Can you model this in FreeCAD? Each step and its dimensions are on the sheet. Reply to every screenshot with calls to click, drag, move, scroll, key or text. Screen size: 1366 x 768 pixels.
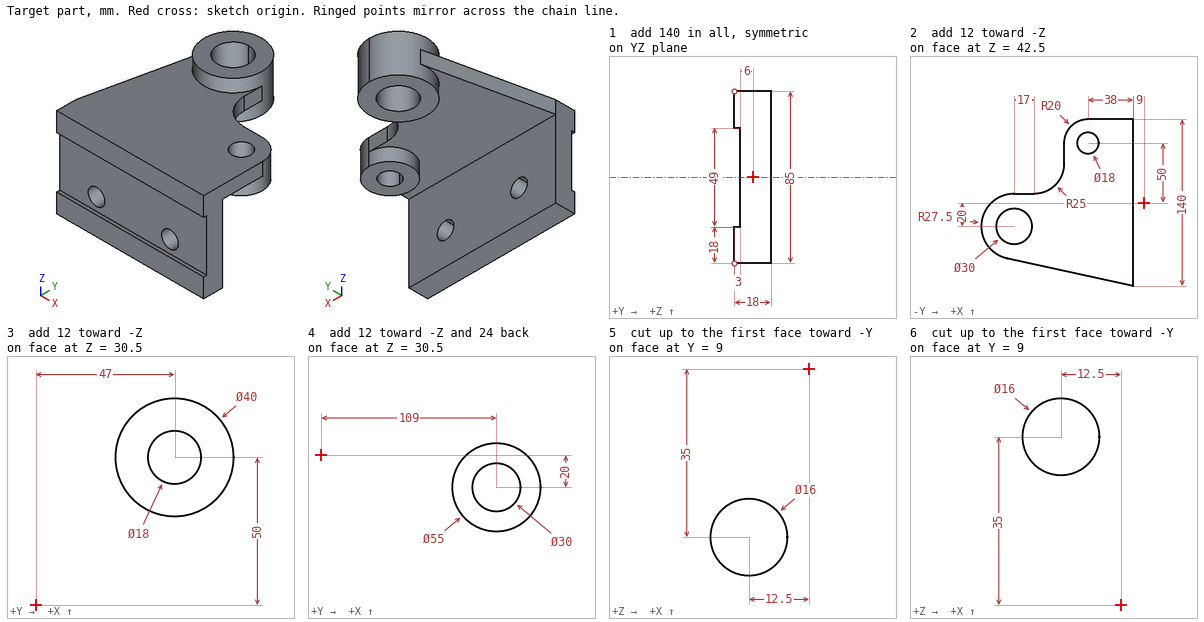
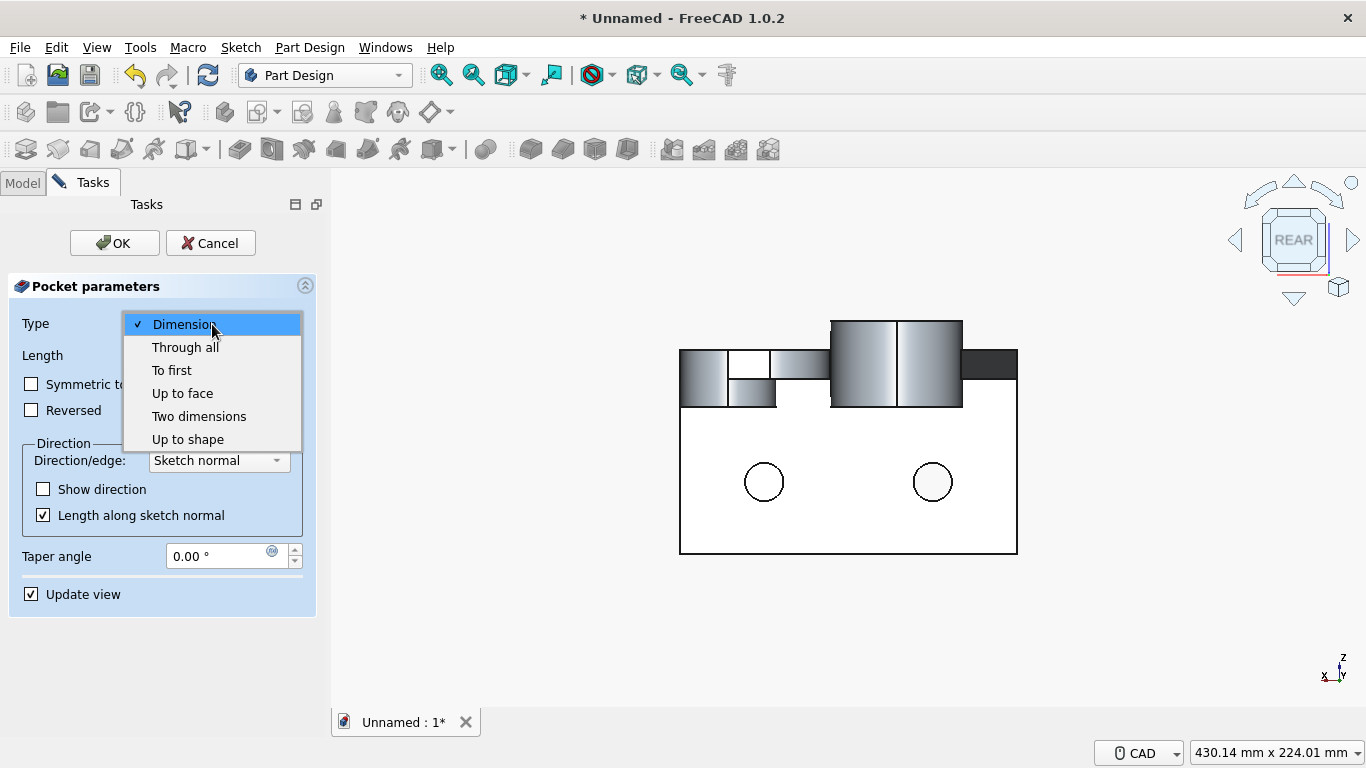
click(212, 370)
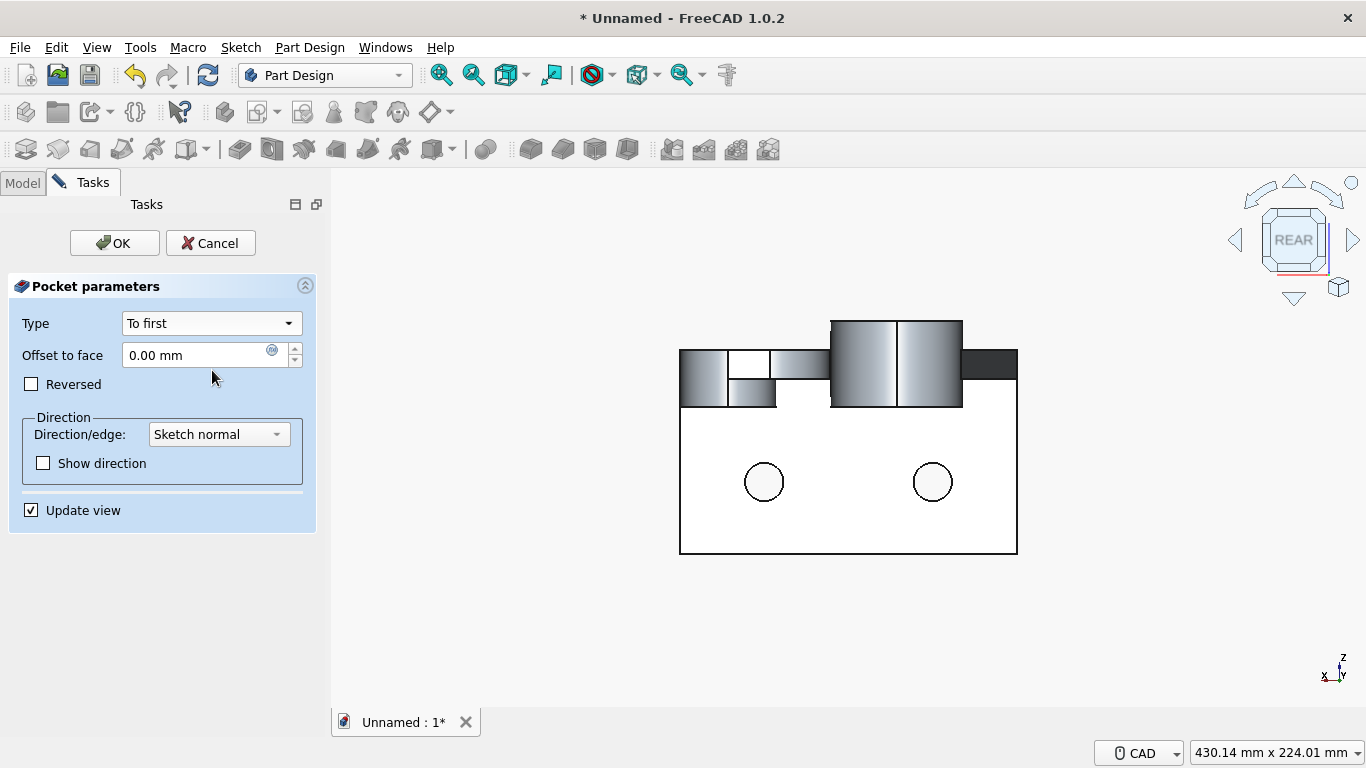
click(115, 243)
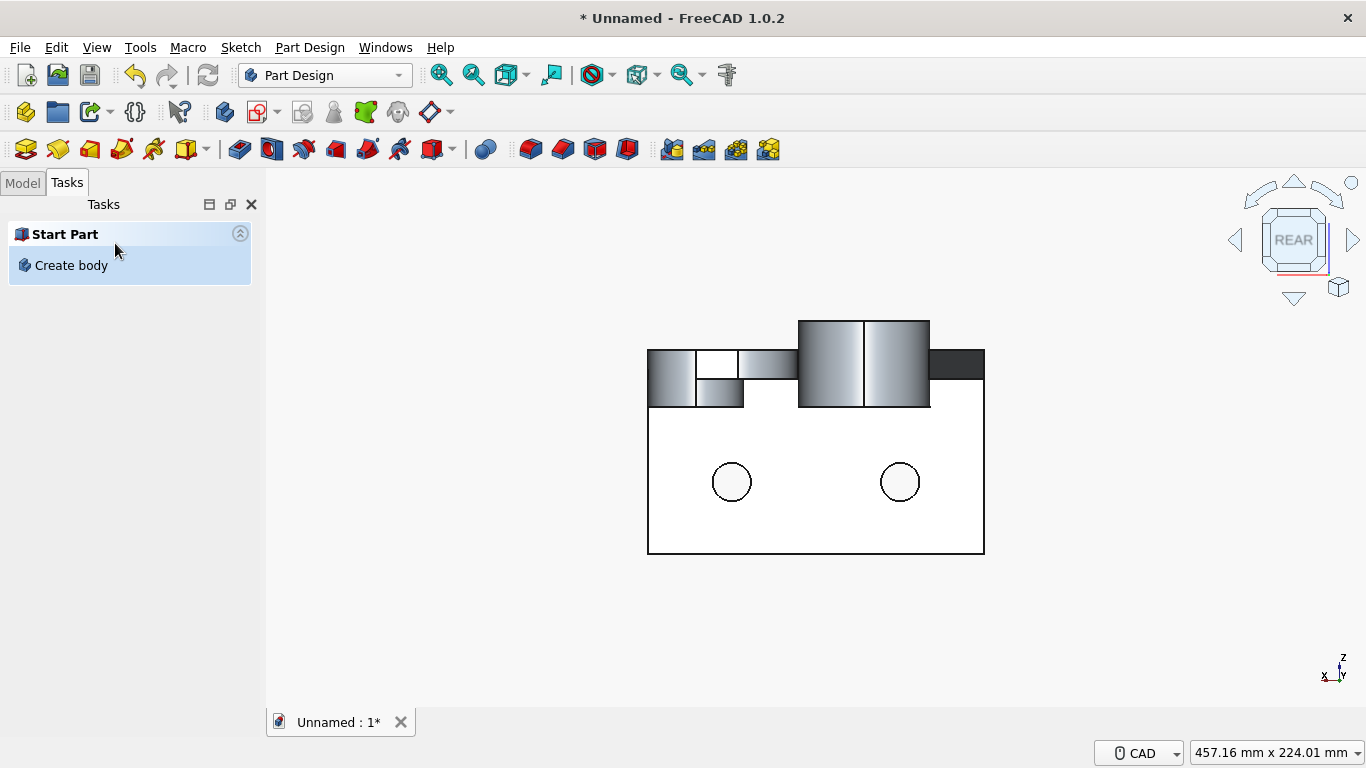
key(v)
key(f)